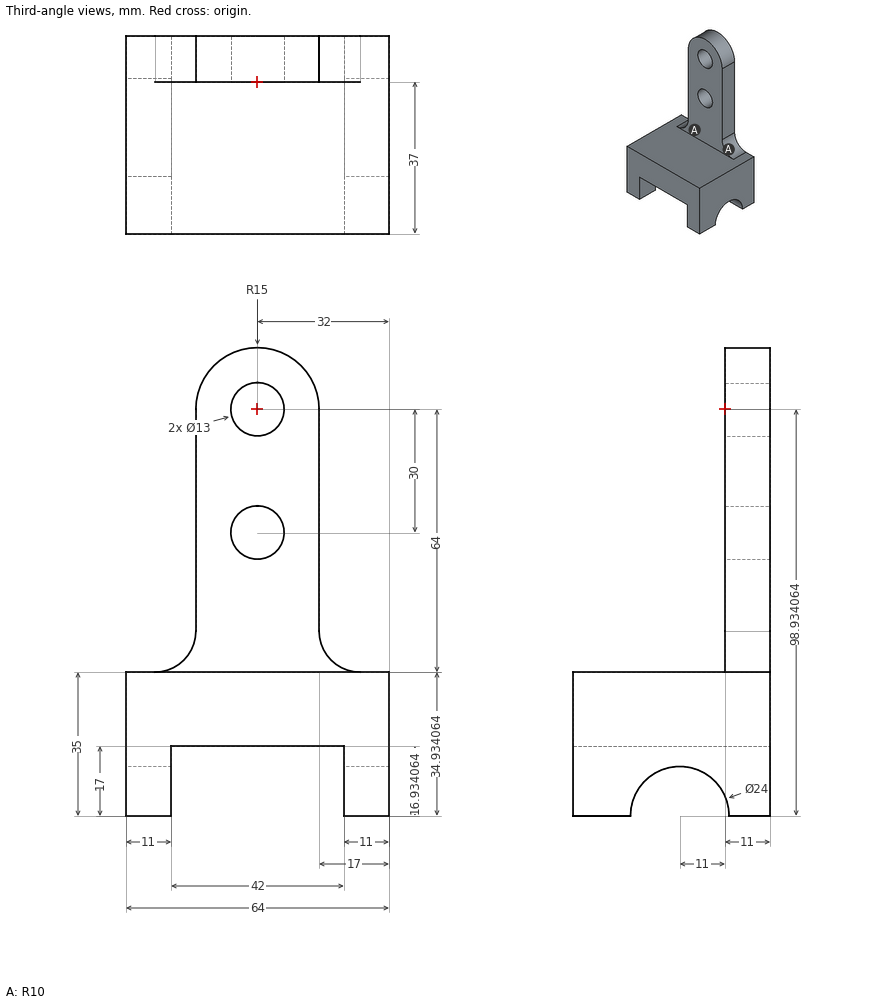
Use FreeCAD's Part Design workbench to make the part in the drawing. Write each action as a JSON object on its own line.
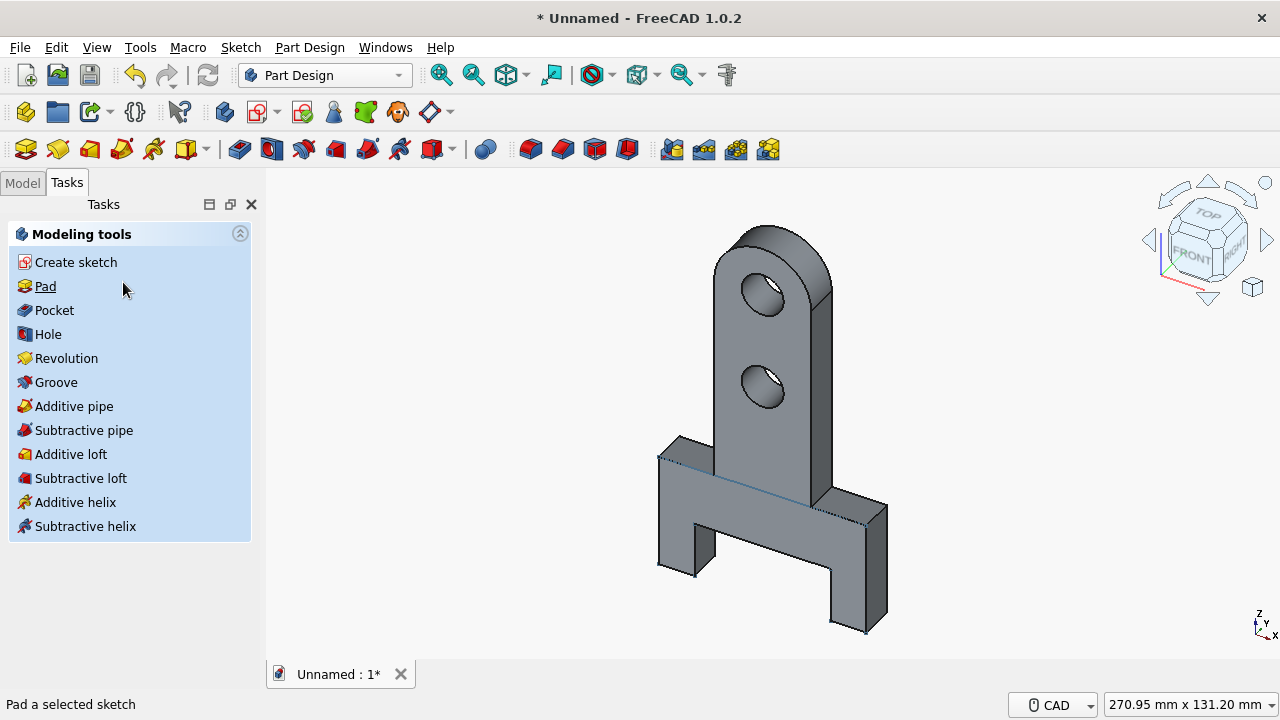
{"action": "left_click", "coordinate": [26, 150]}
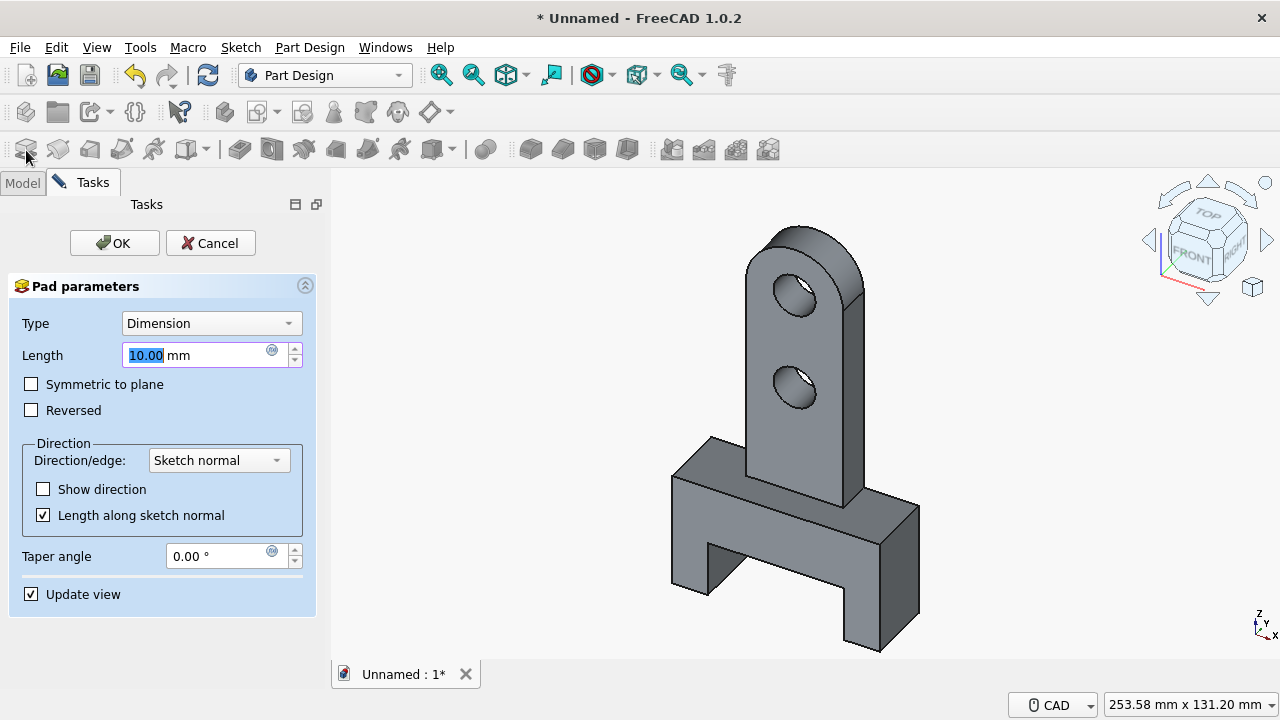
{"action": "type", "text": "37"}
{"action": "key", "text": "Tab"}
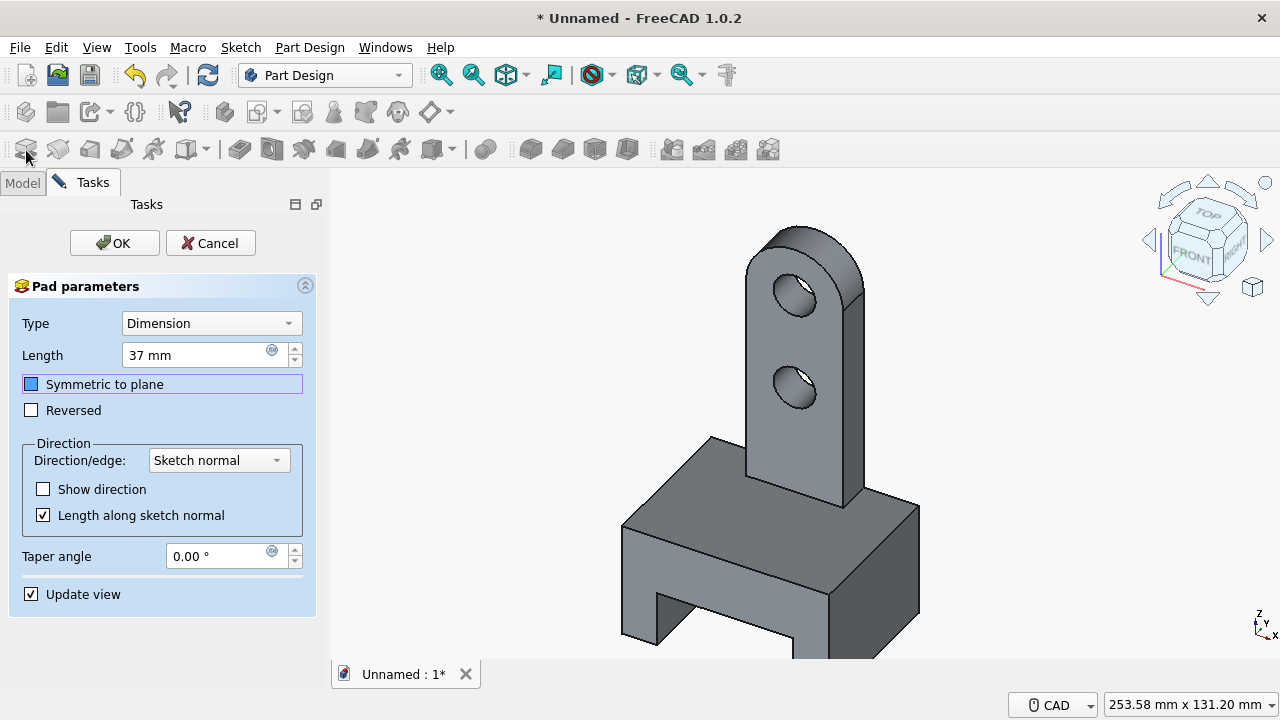
{"action": "left_click", "coordinate": [115, 243]}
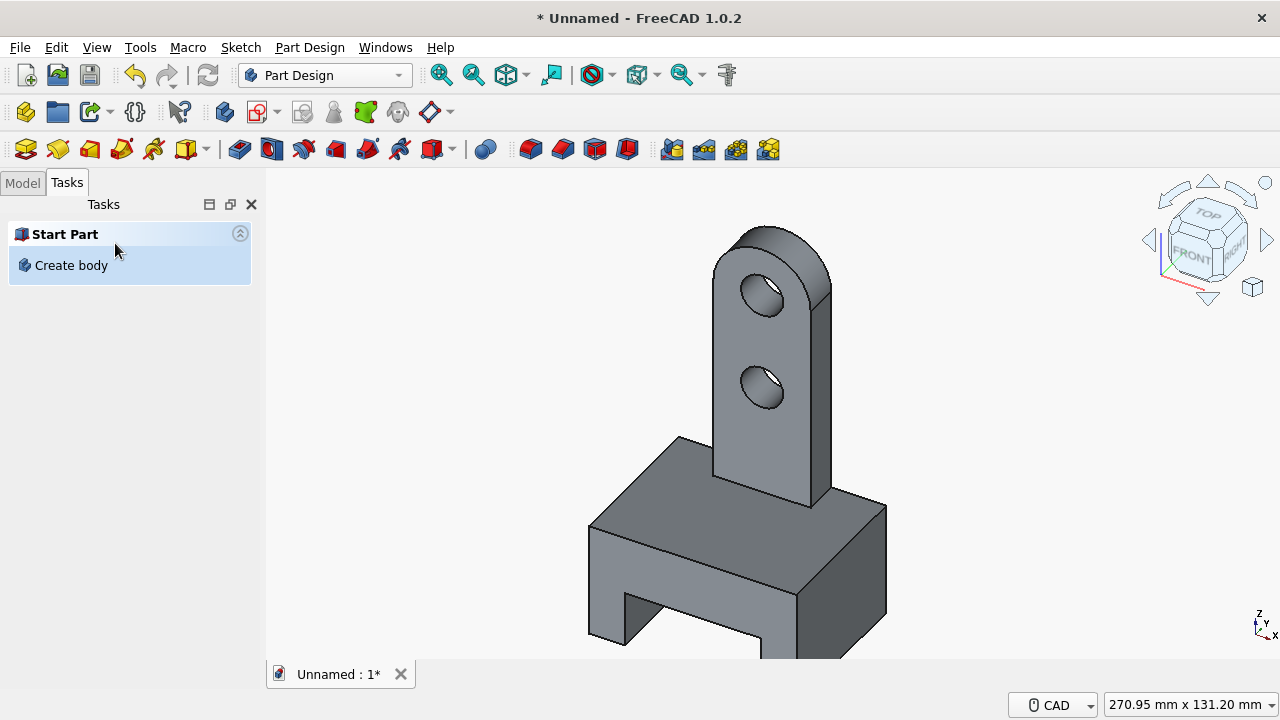
{"action": "left_click", "coordinate": [442, 76]}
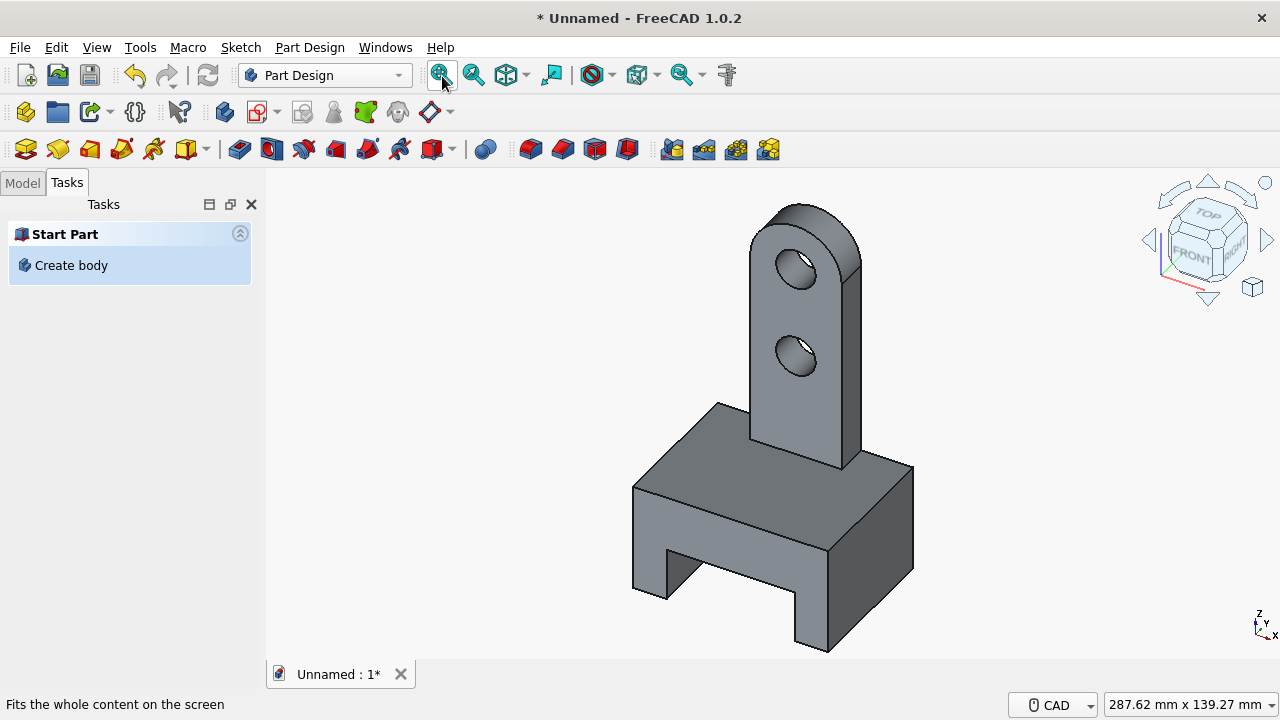
{"action": "key", "text": "0"}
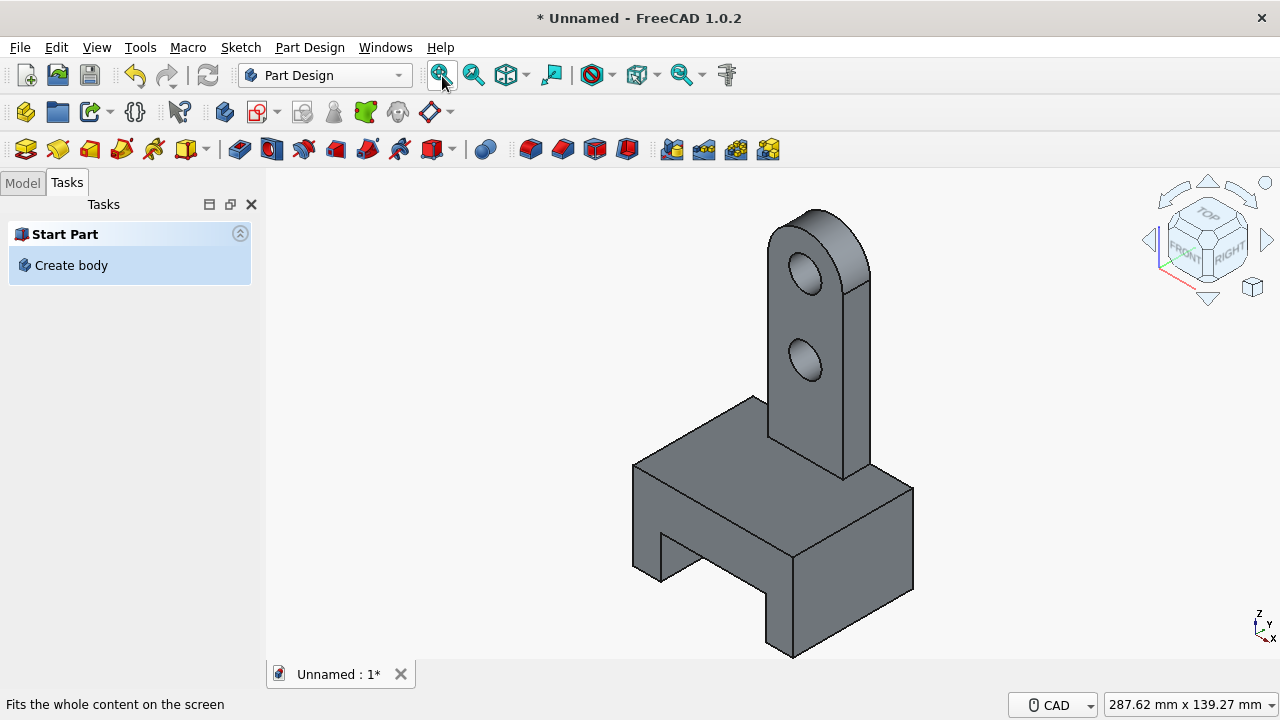
{"action": "key", "text": "2"}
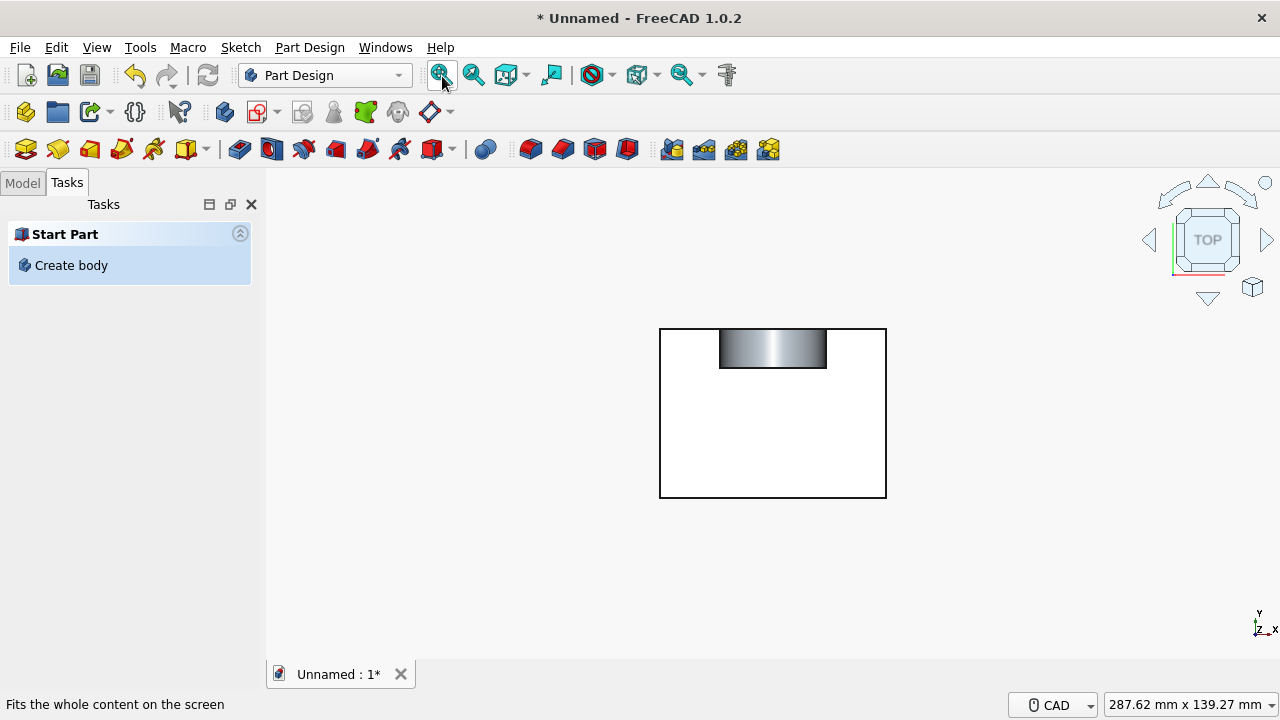
{"action": "left_click", "coordinate": [442, 76]}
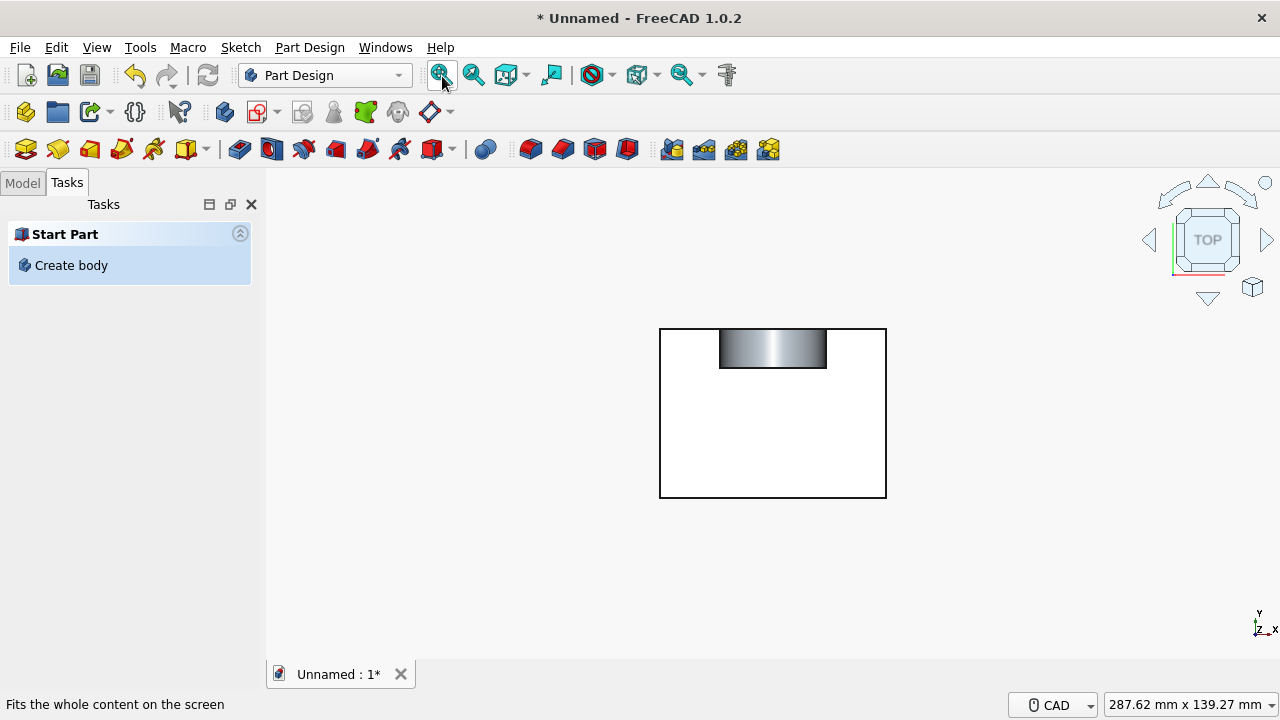
{"action": "key", "text": "1"}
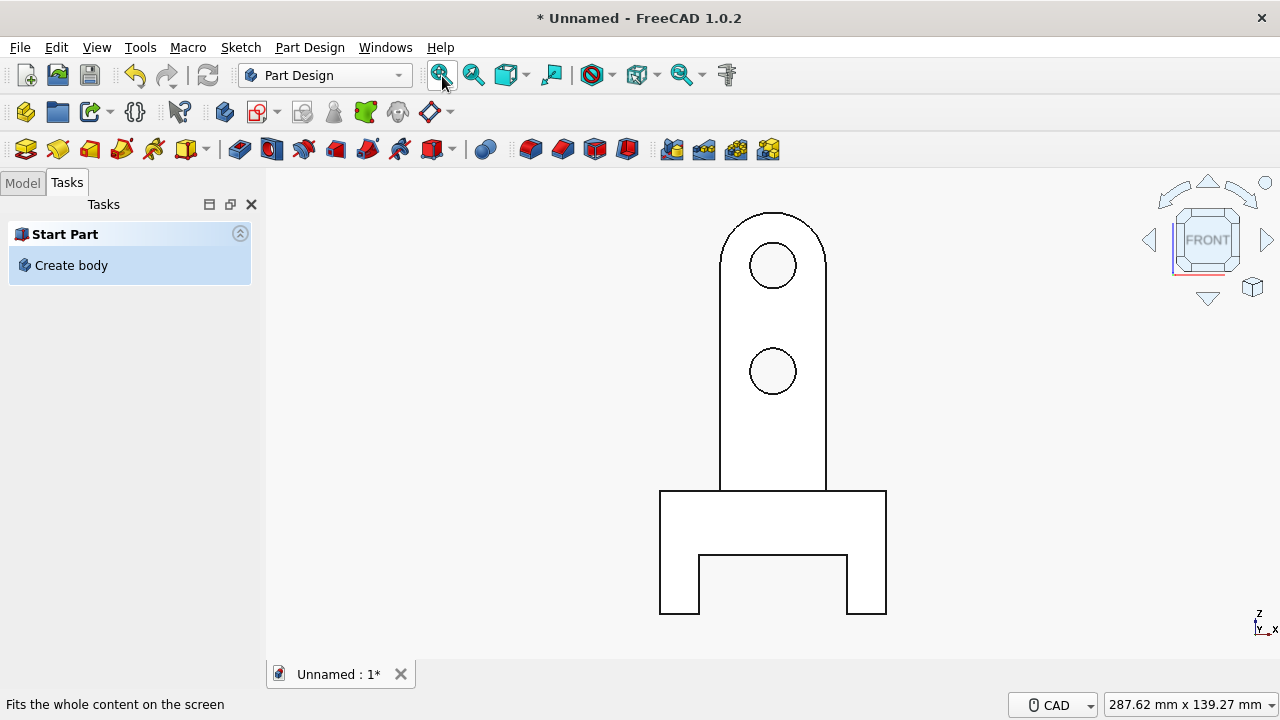
{"action": "key", "text": "3"}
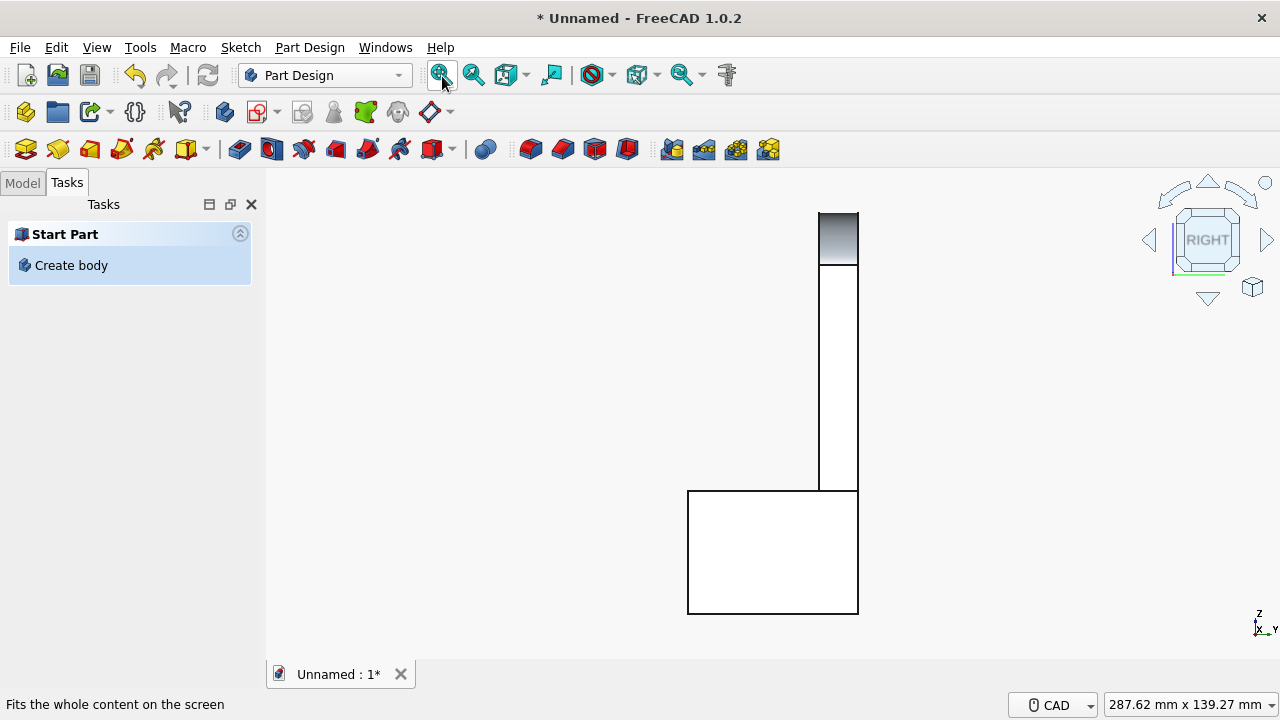
{"action": "key", "text": "5"}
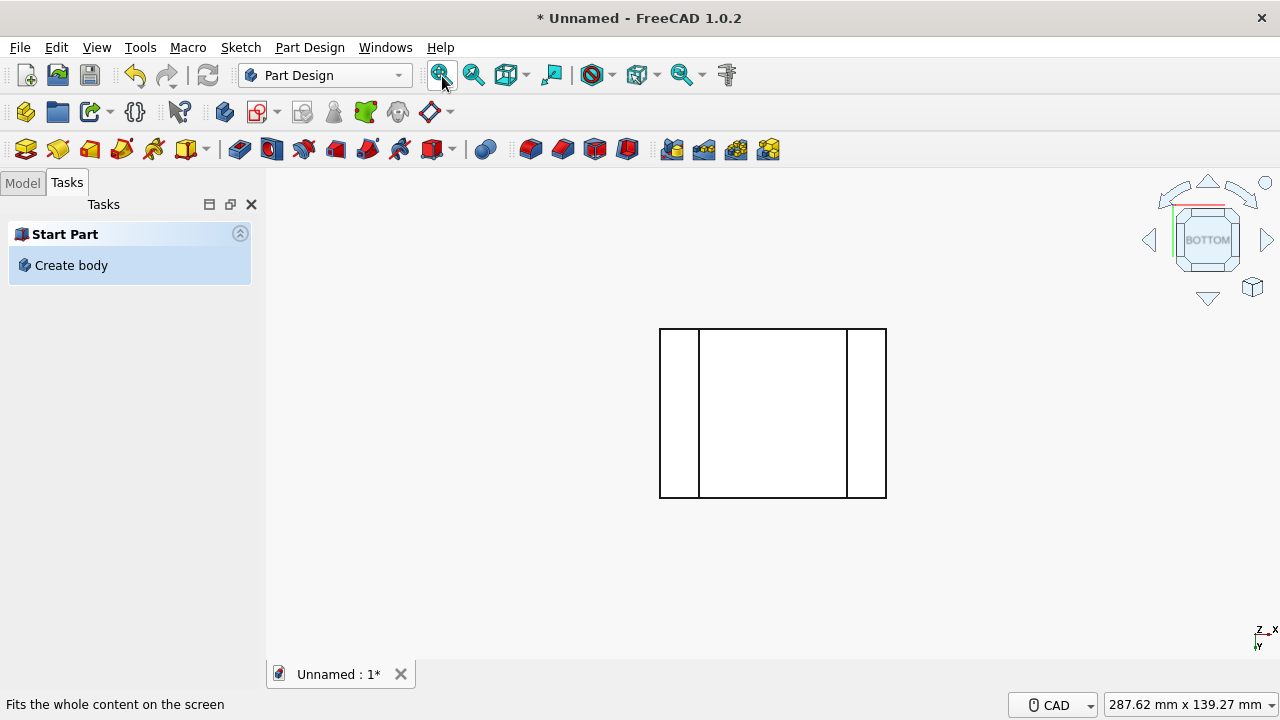
{"action": "left_click", "coordinate": [442, 76]}